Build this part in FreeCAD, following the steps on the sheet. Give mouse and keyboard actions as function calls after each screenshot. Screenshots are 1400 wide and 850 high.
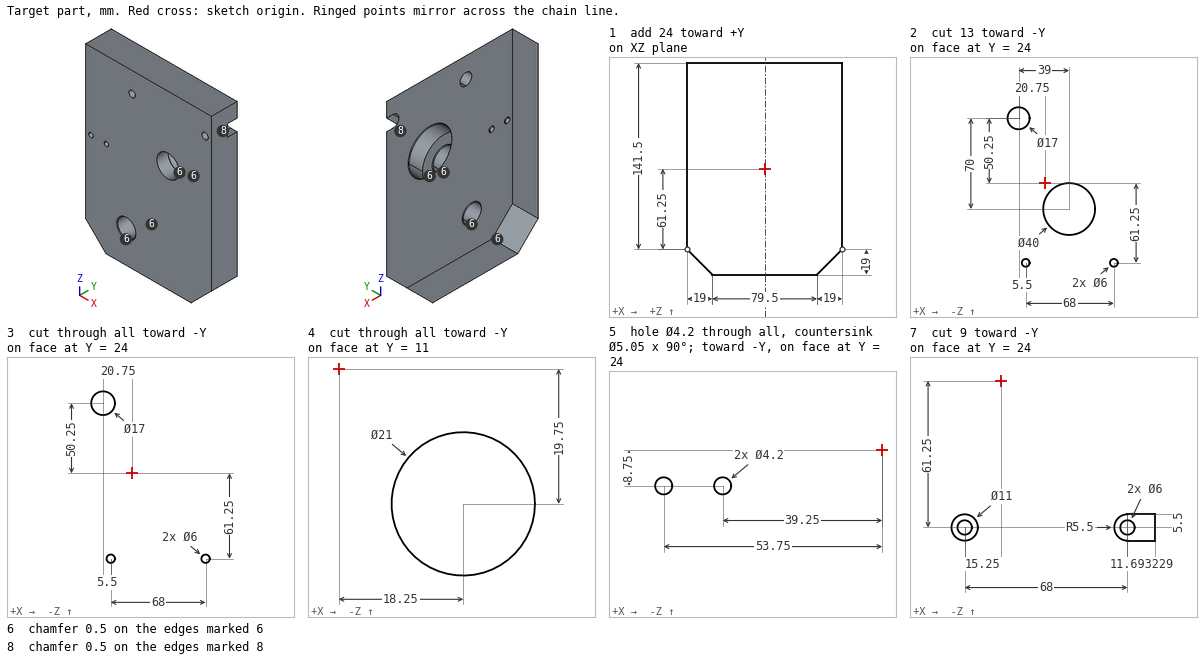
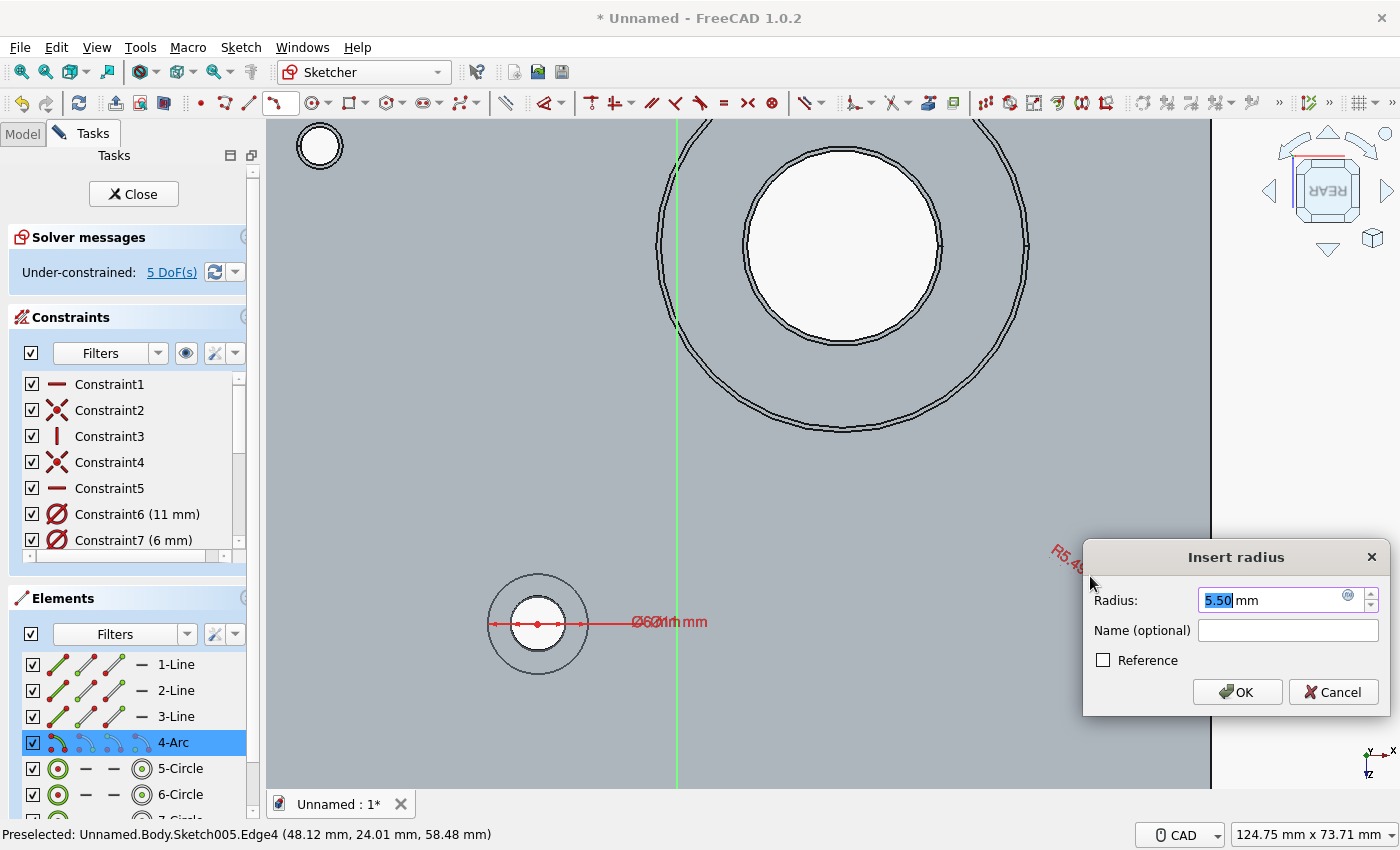
text(5.5)
key(Return)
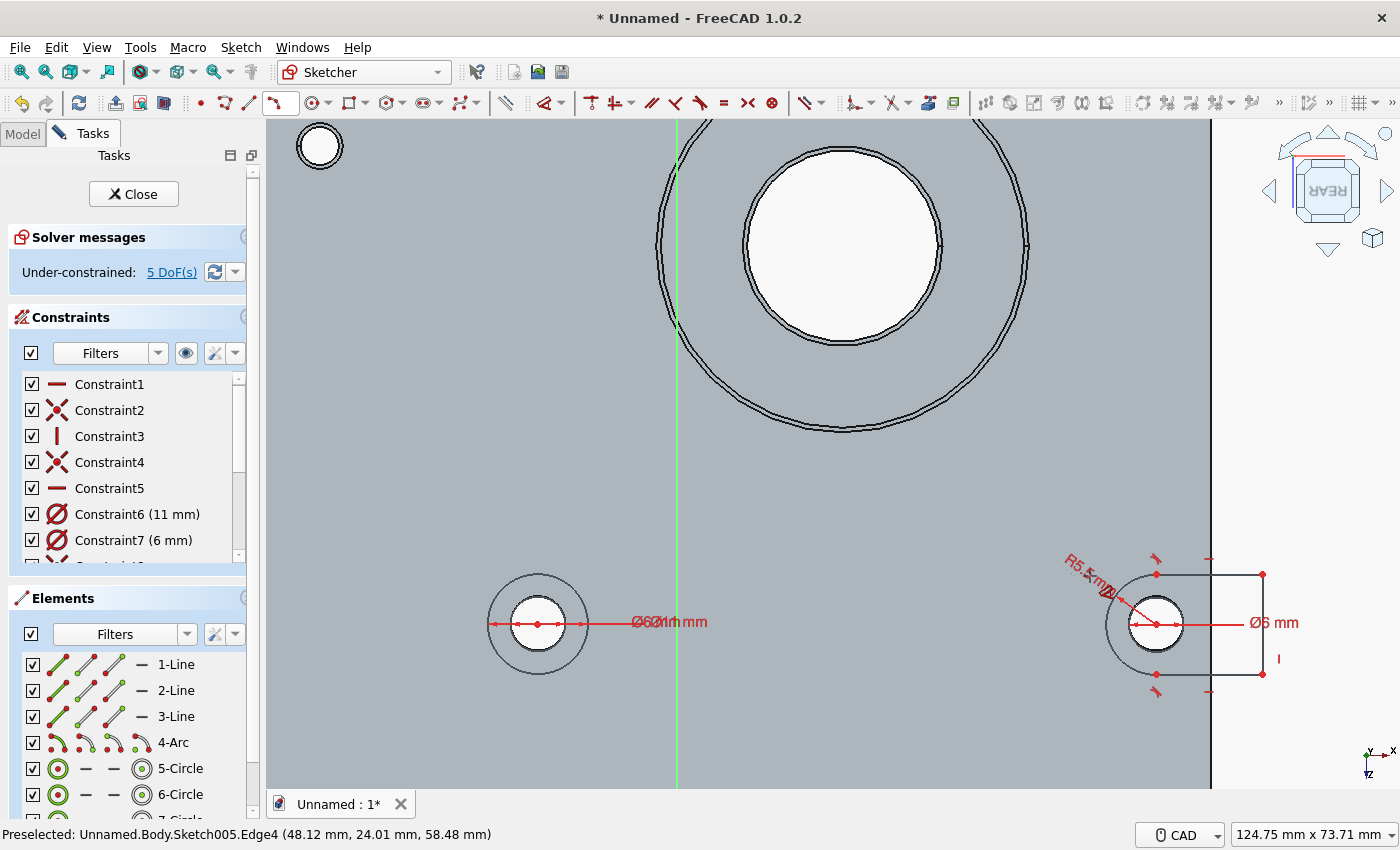
click(1156, 575)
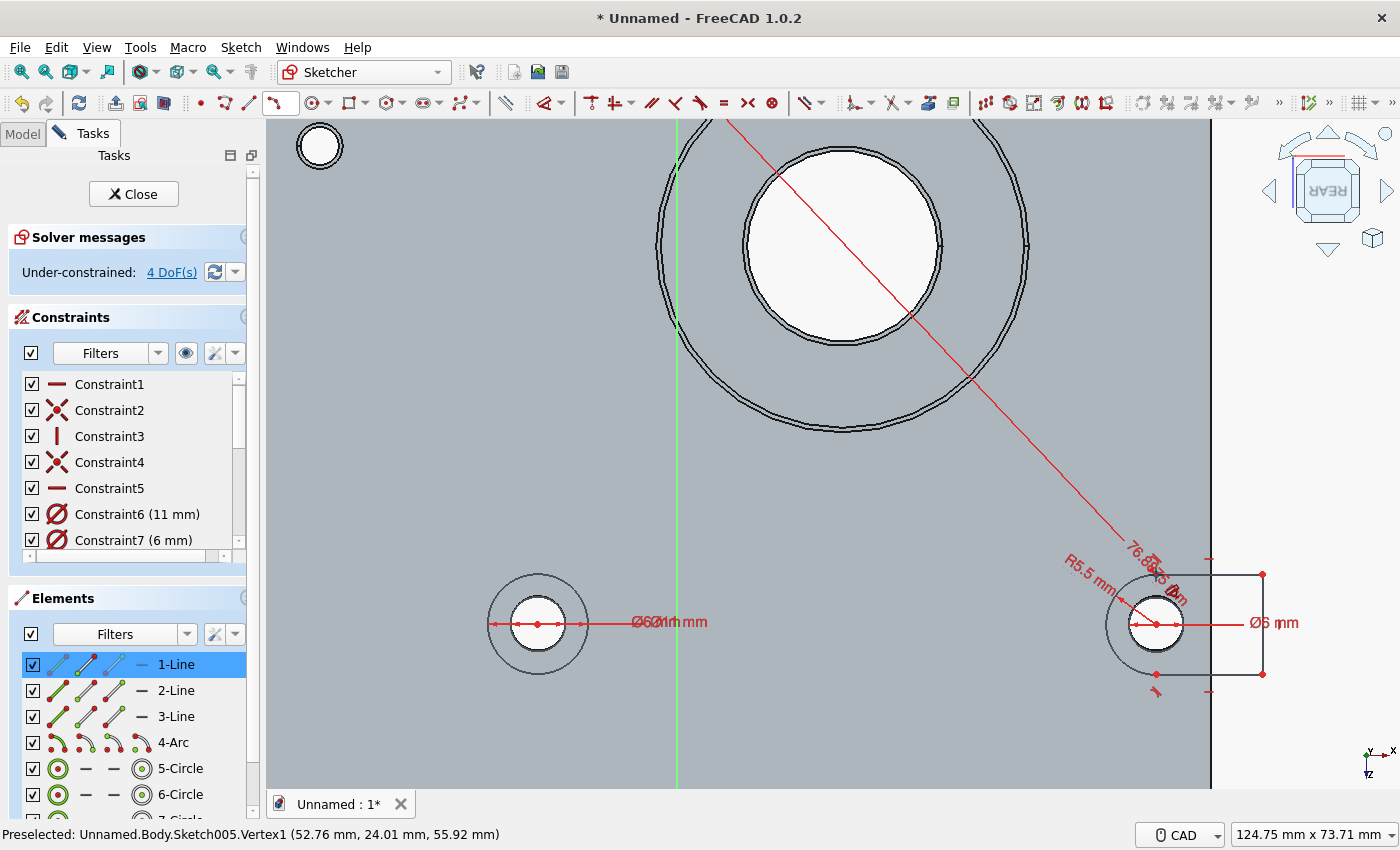
click(538, 624)
click(847, 658)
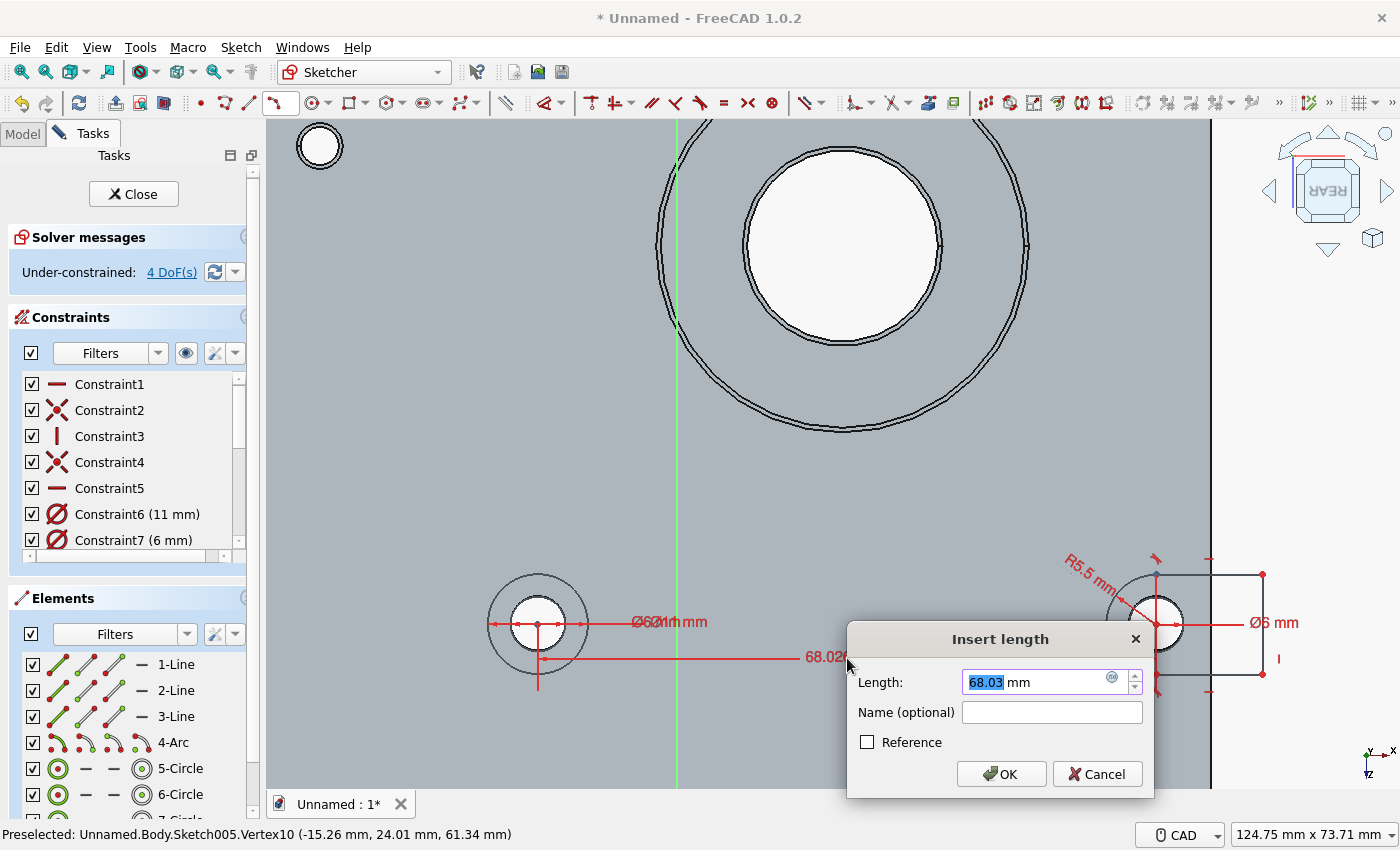
text(68)
key(Return)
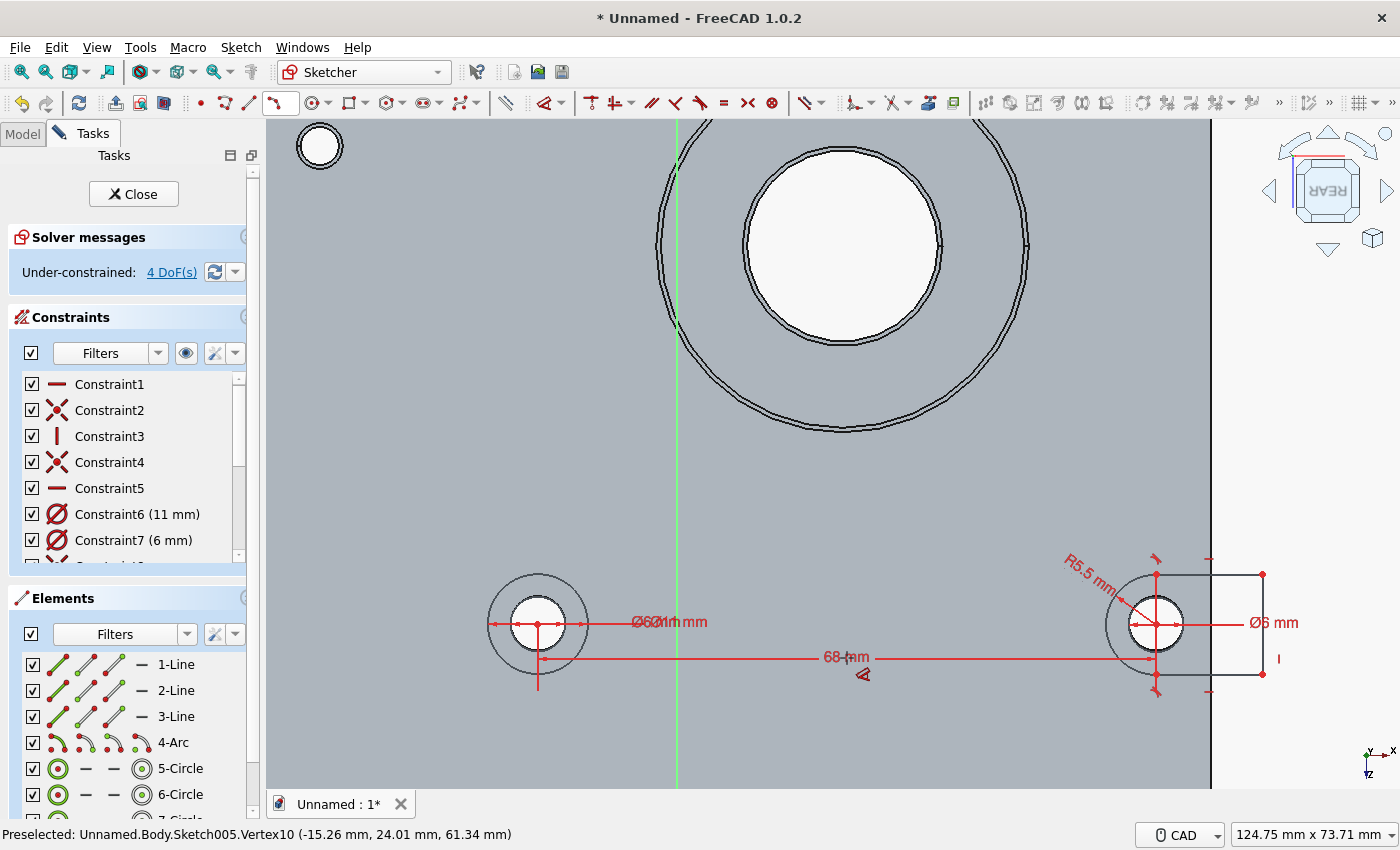
click(1156, 575)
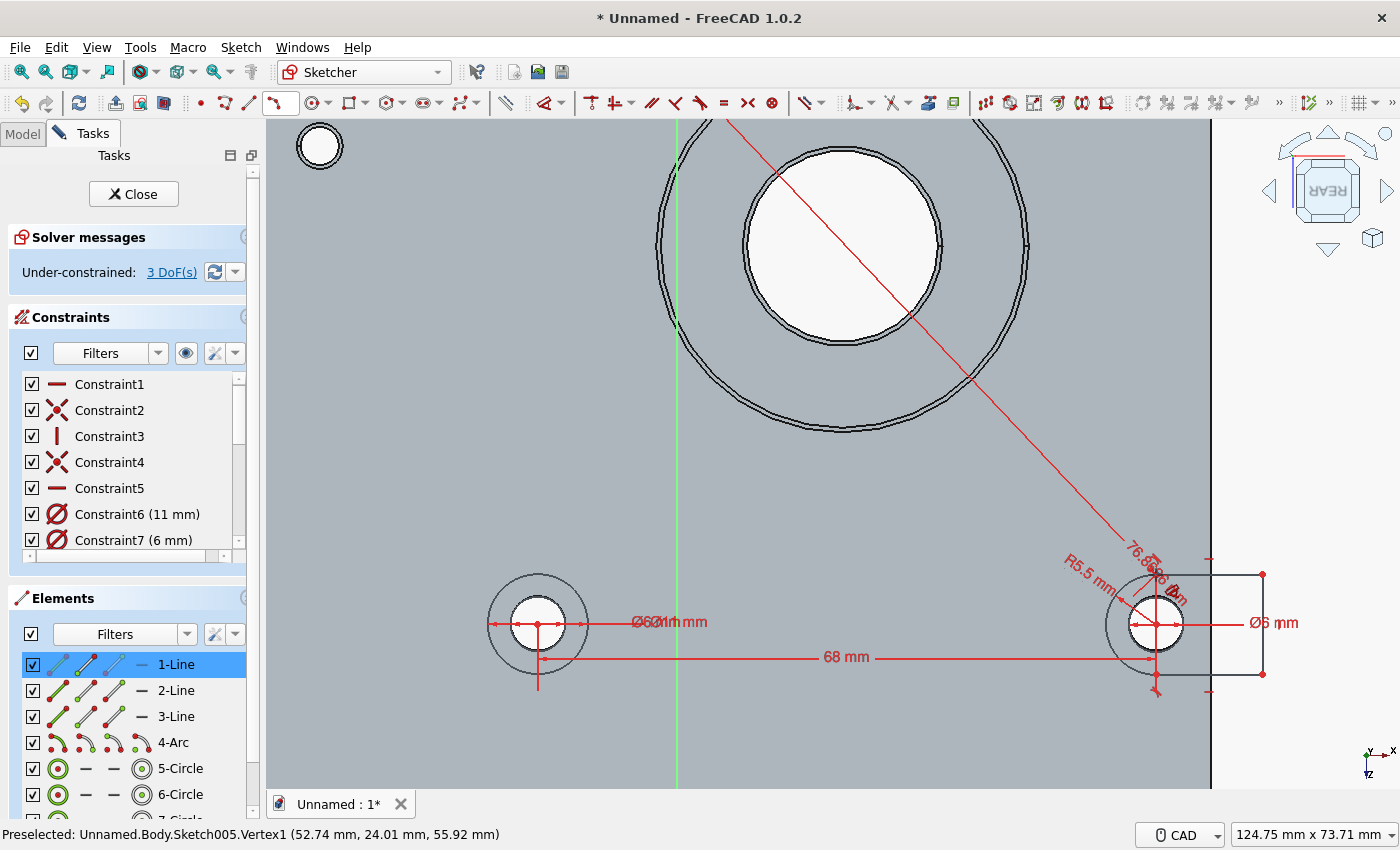
click(538, 624)
click(1190, 599)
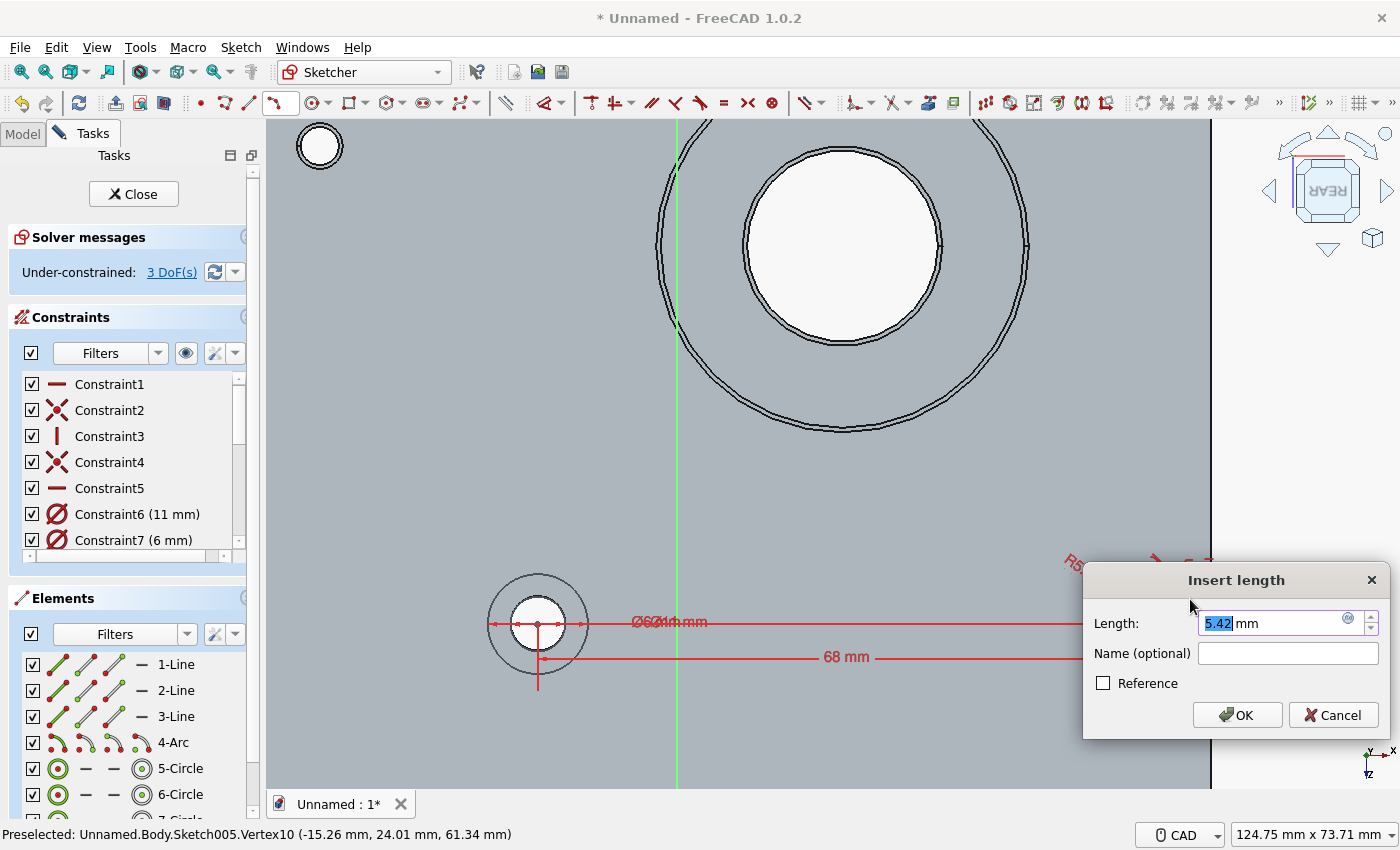
text(5.5)
key(Return)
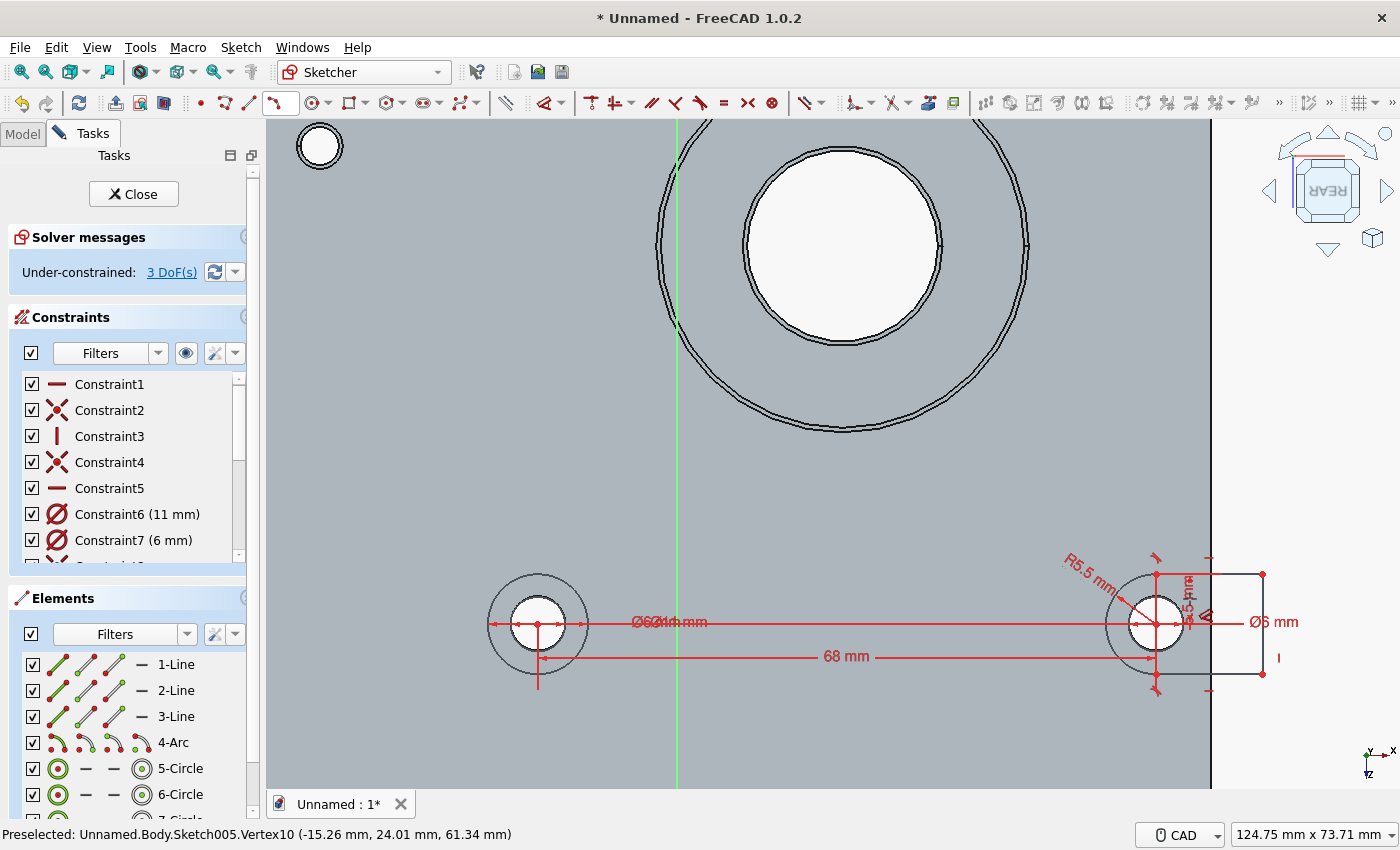
click(538, 624)
click(607, 658)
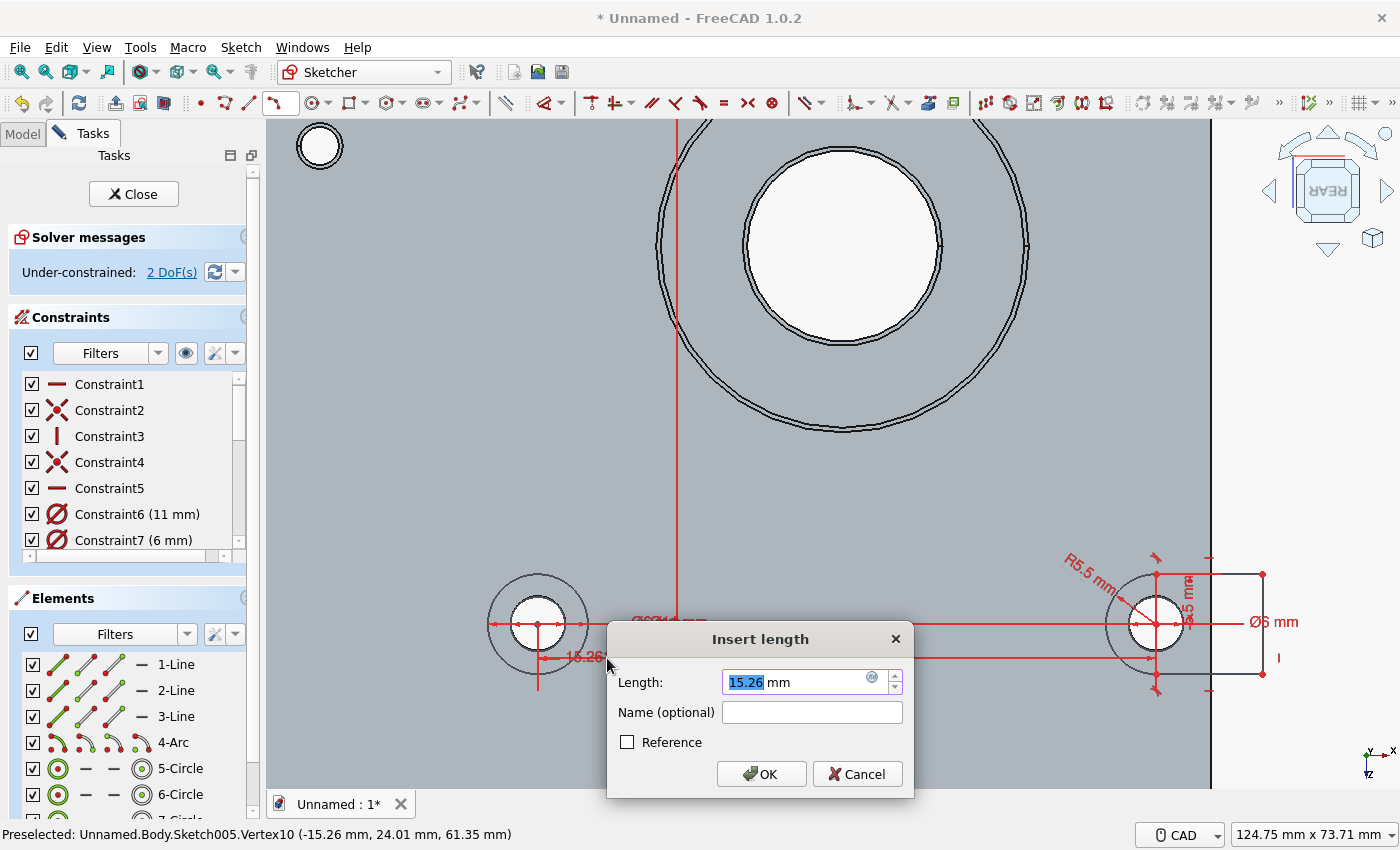
text(15.25)
key(Return)